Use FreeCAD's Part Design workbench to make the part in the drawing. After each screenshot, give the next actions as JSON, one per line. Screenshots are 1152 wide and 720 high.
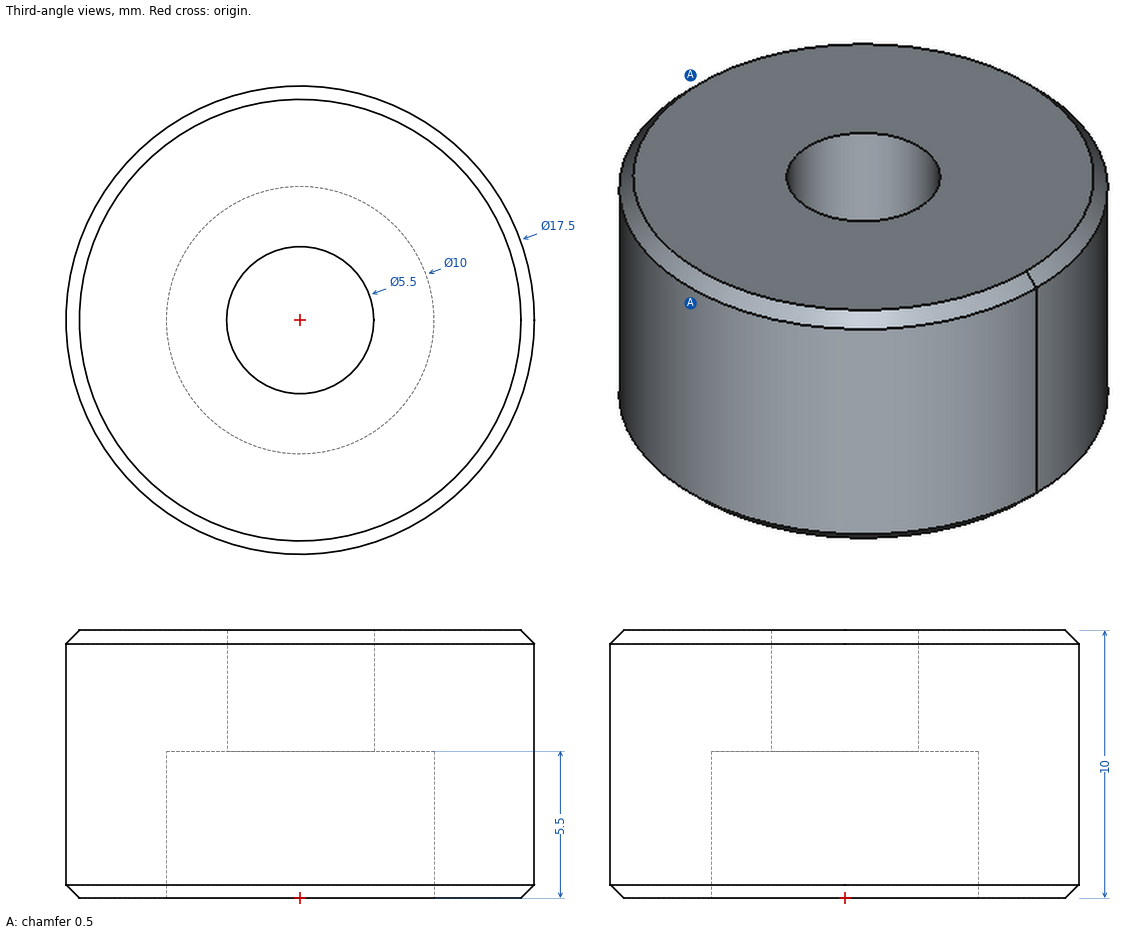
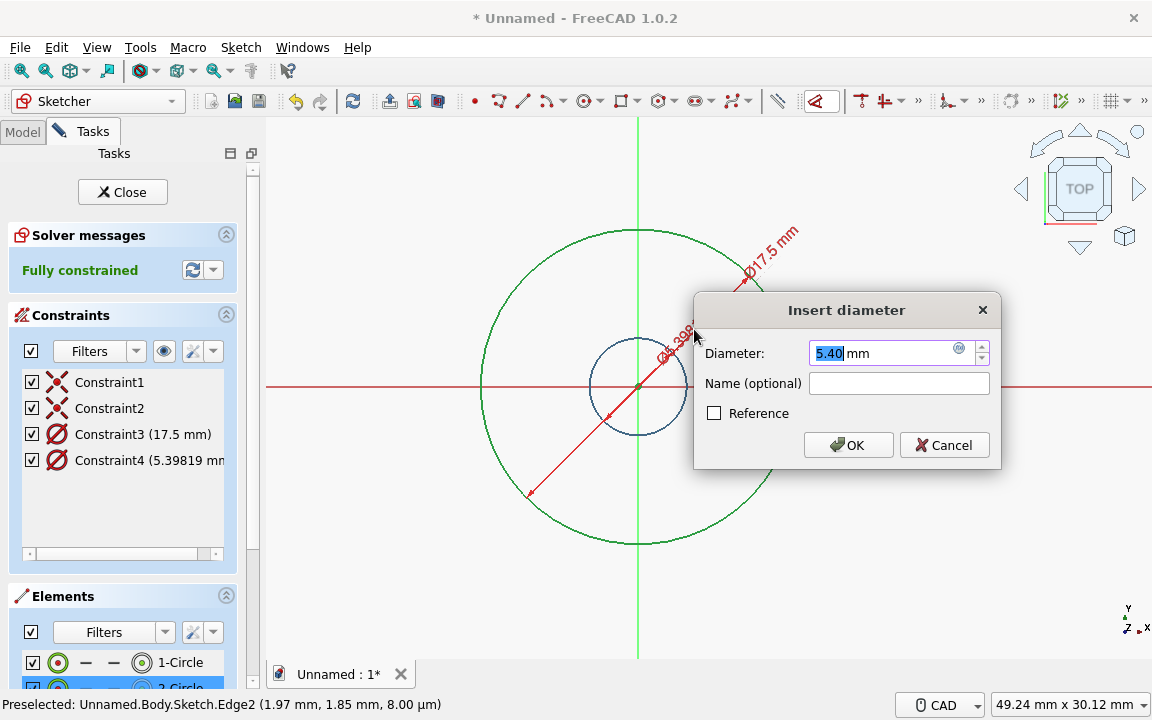
{"action": "type", "text": "5.5"}
{"action": "key", "text": "Return"}
{"action": "key", "text": "Escape"}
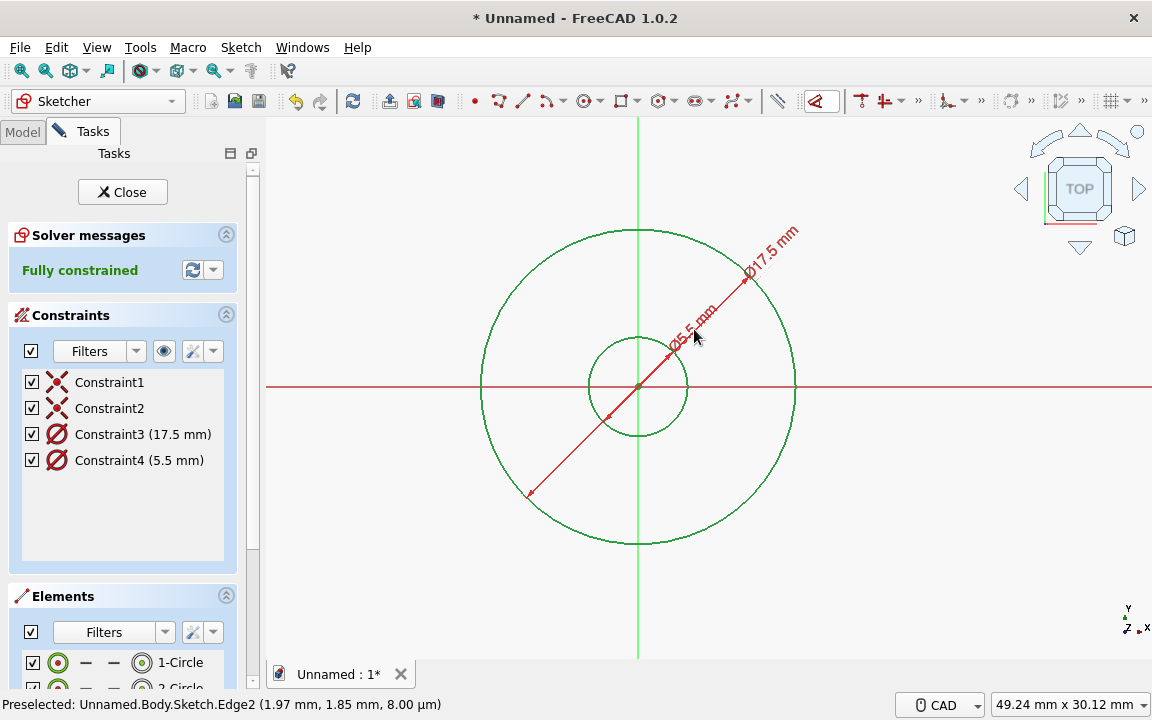
{"action": "left_click", "coordinate": [123, 192]}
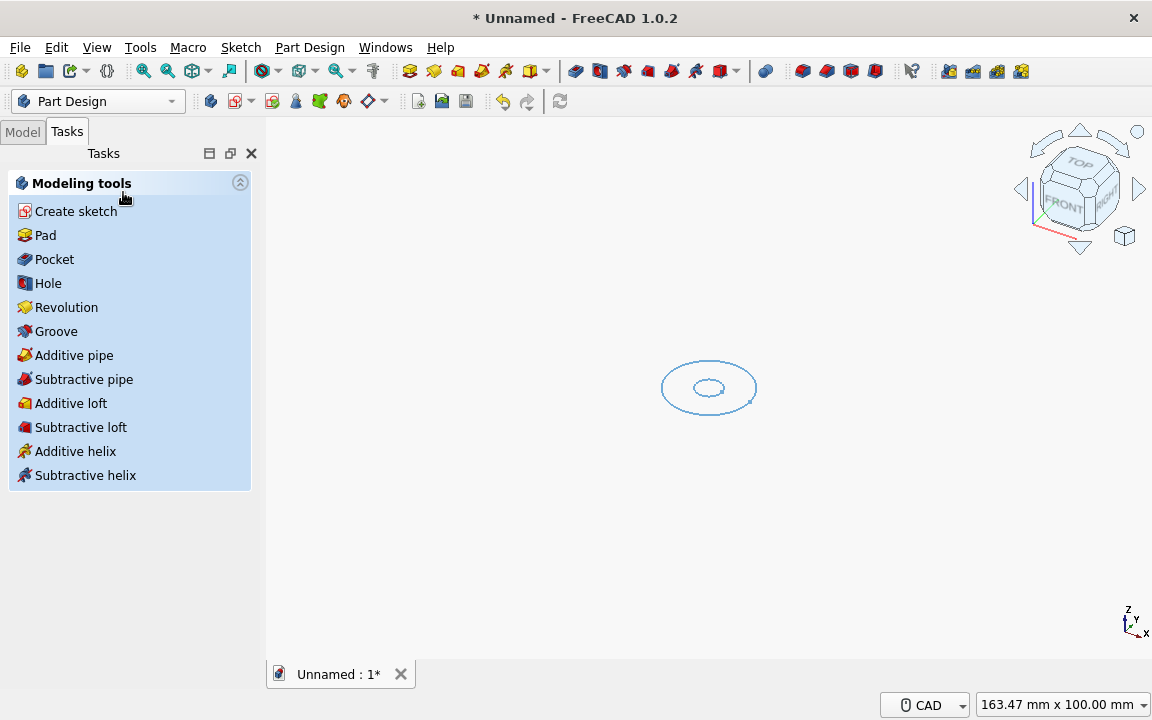
{"action": "left_click", "coordinate": [410, 72]}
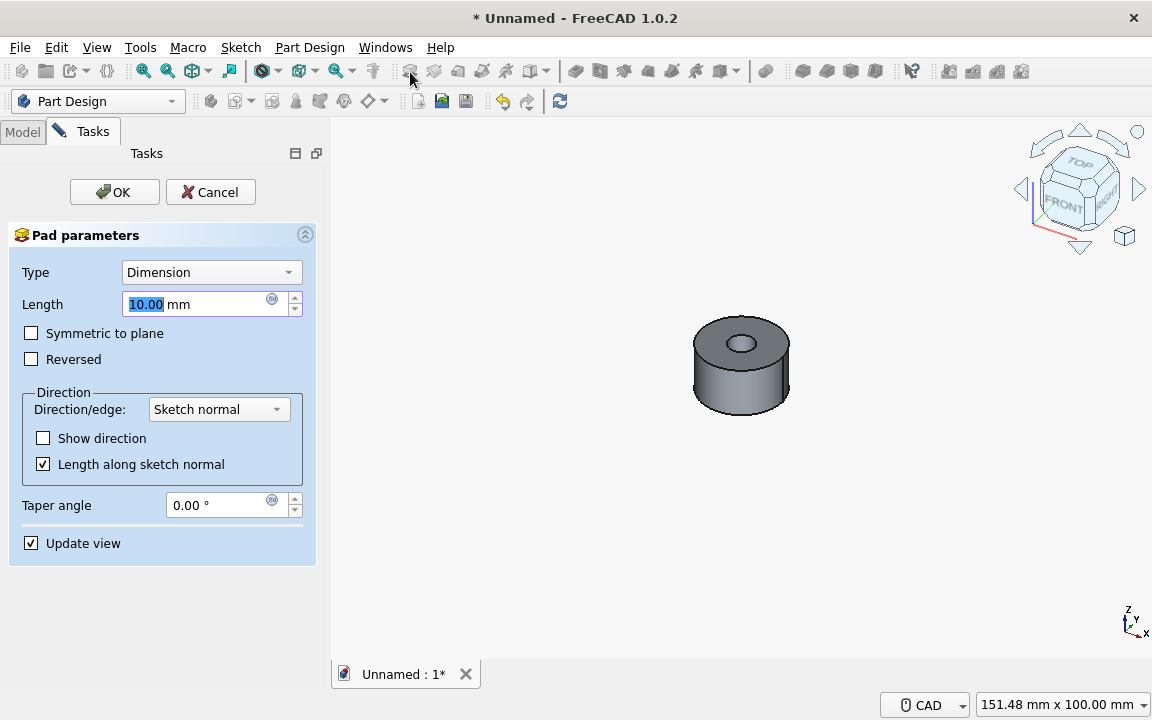
{"action": "type", "text": "10"}
{"action": "key", "text": "Tab"}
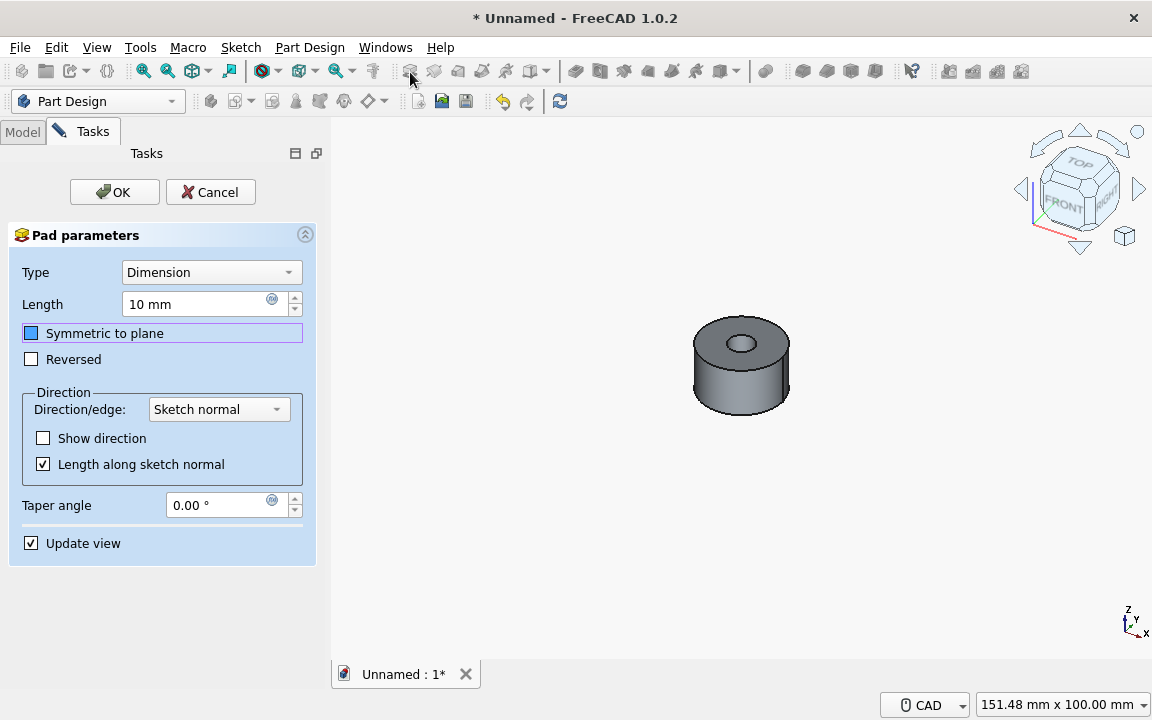
{"action": "left_click", "coordinate": [115, 192]}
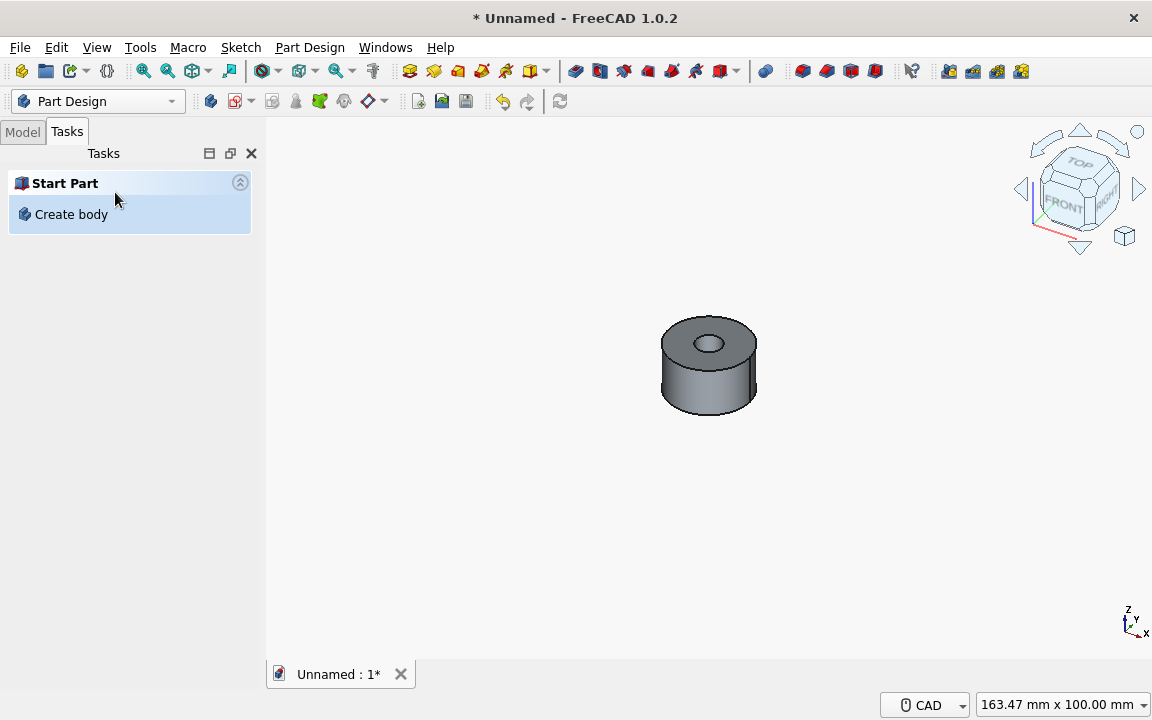
{"action": "key", "text": "v f"}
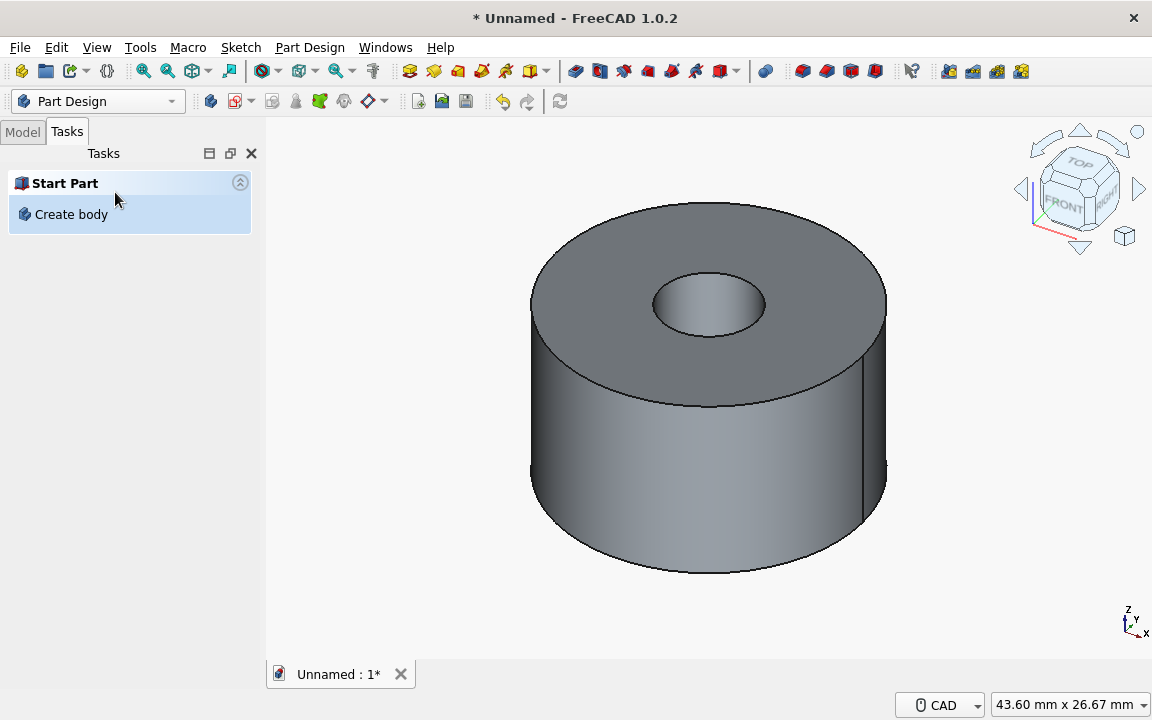
{"action": "left_click", "coordinate": [236, 102]}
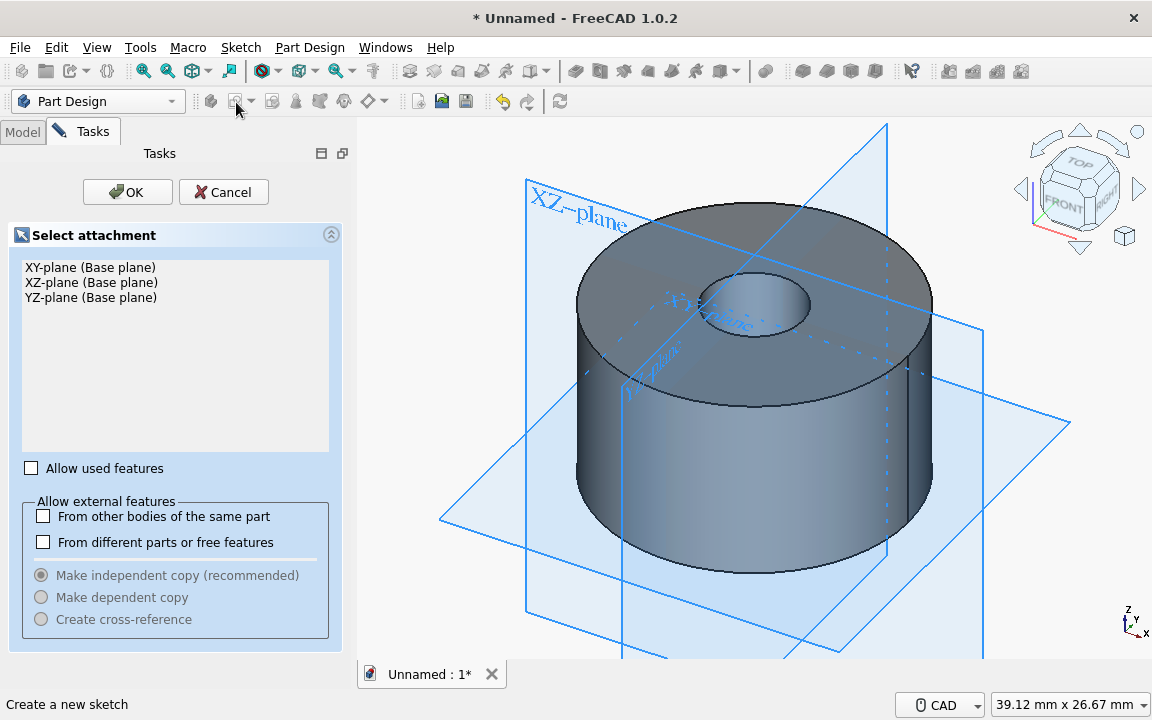
{"action": "left_click", "coordinate": [82, 268]}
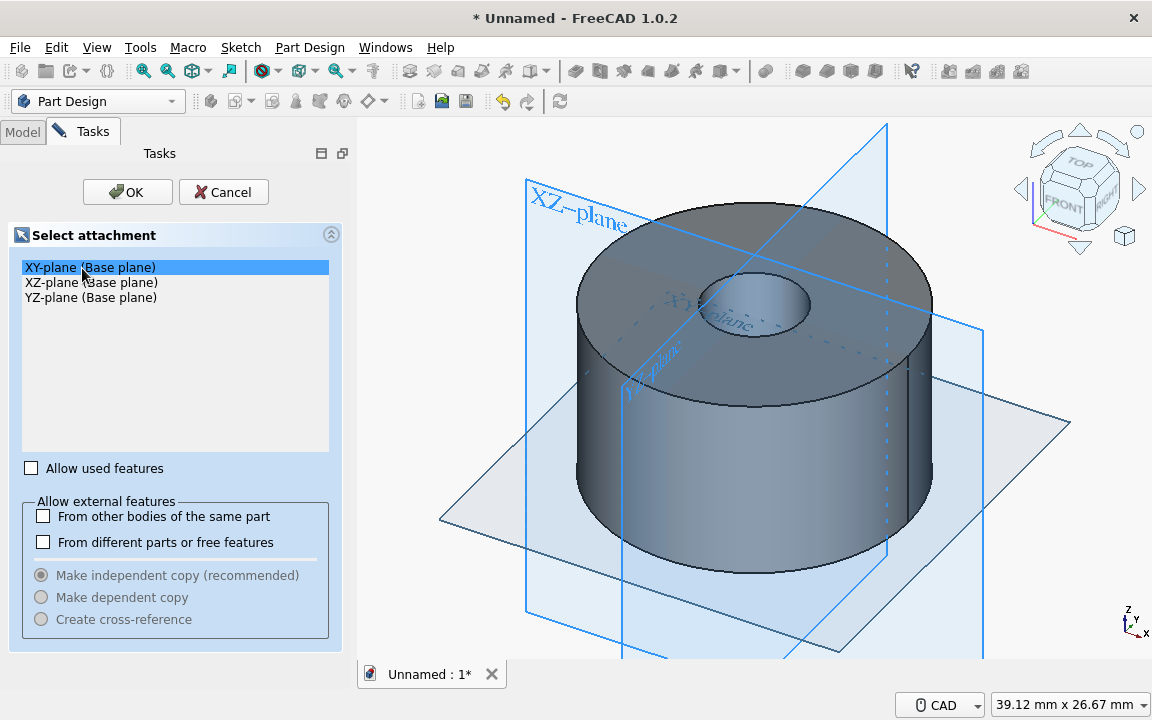
{"action": "left_click", "coordinate": [128, 192]}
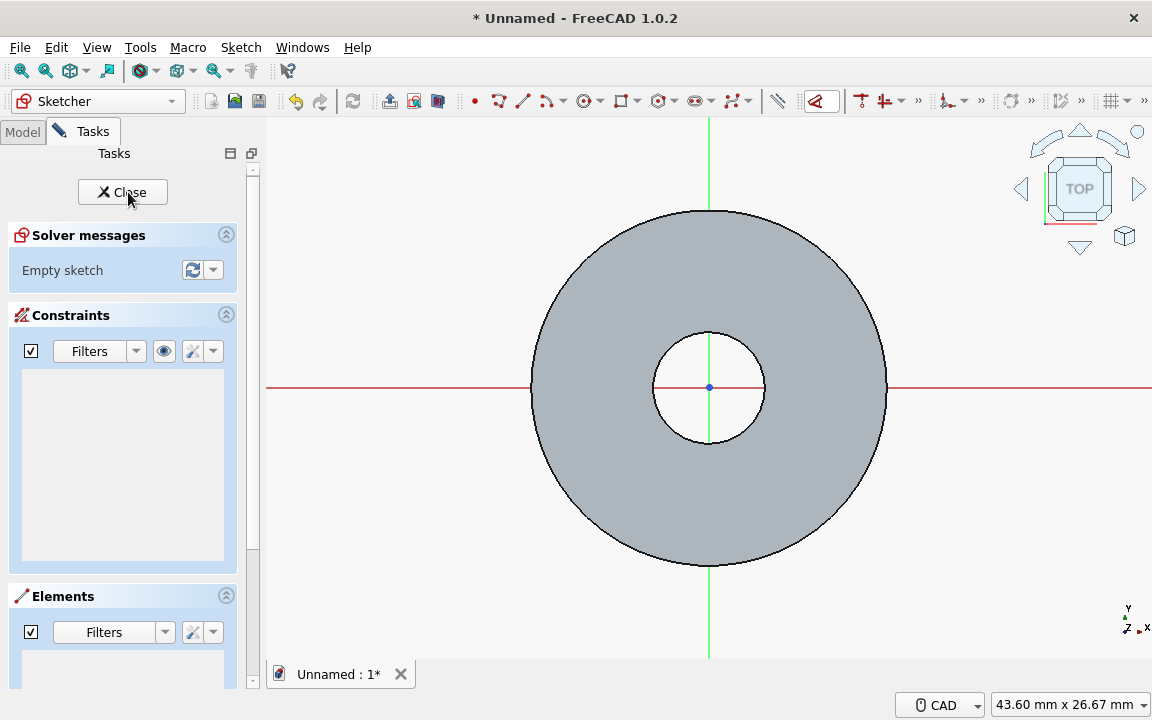
{"action": "key", "text": "q s"}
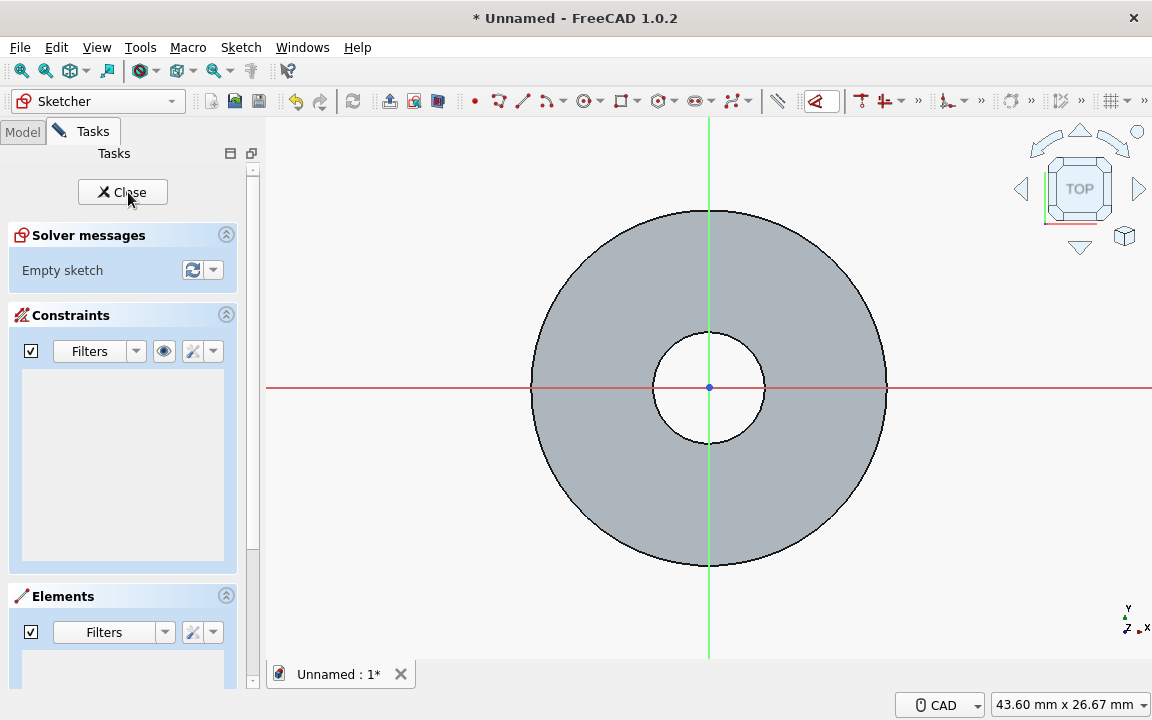
{"action": "scroll", "coordinate": [792, 388], "scroll_direction": "up", "scroll_amount": 3}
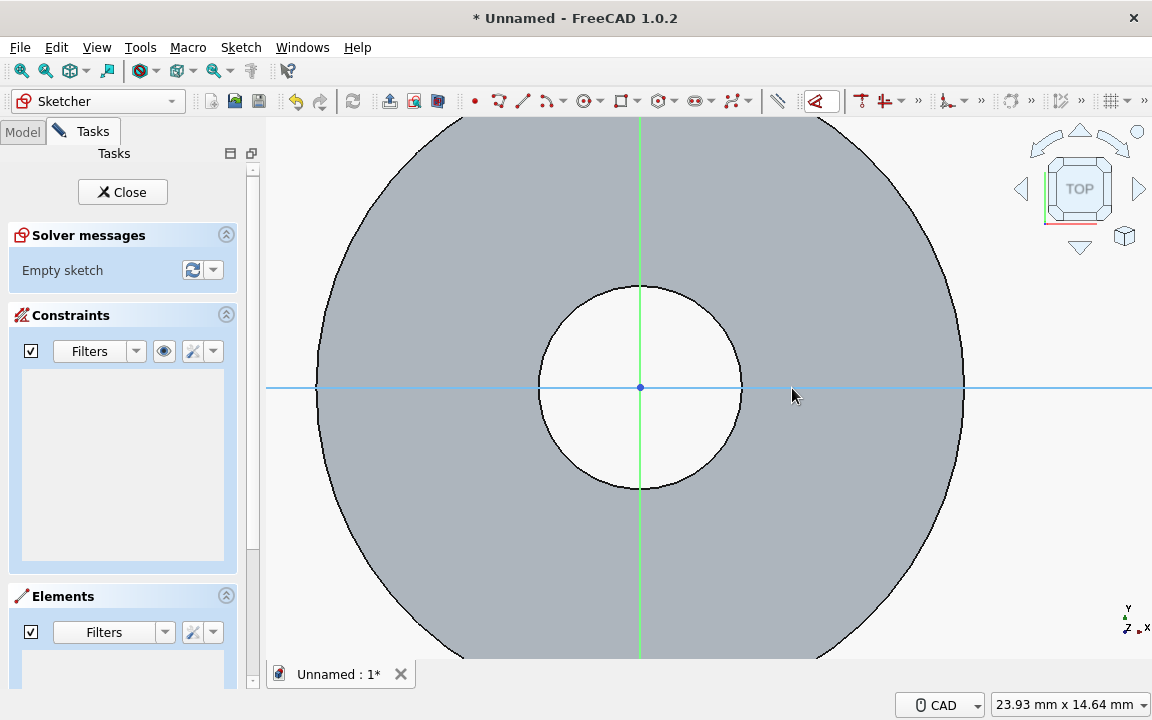
{"action": "key", "text": "g c"}